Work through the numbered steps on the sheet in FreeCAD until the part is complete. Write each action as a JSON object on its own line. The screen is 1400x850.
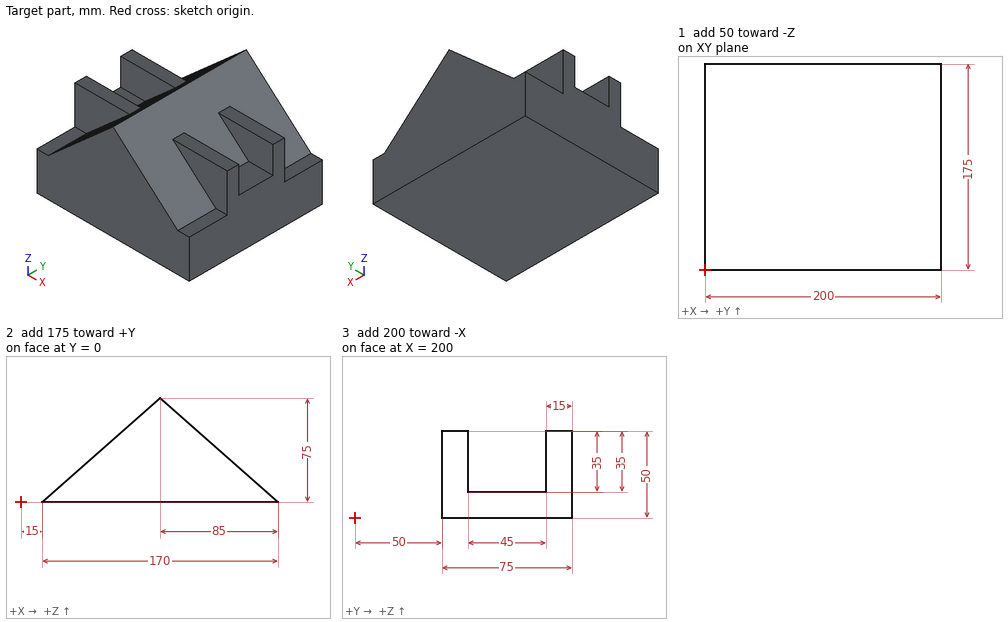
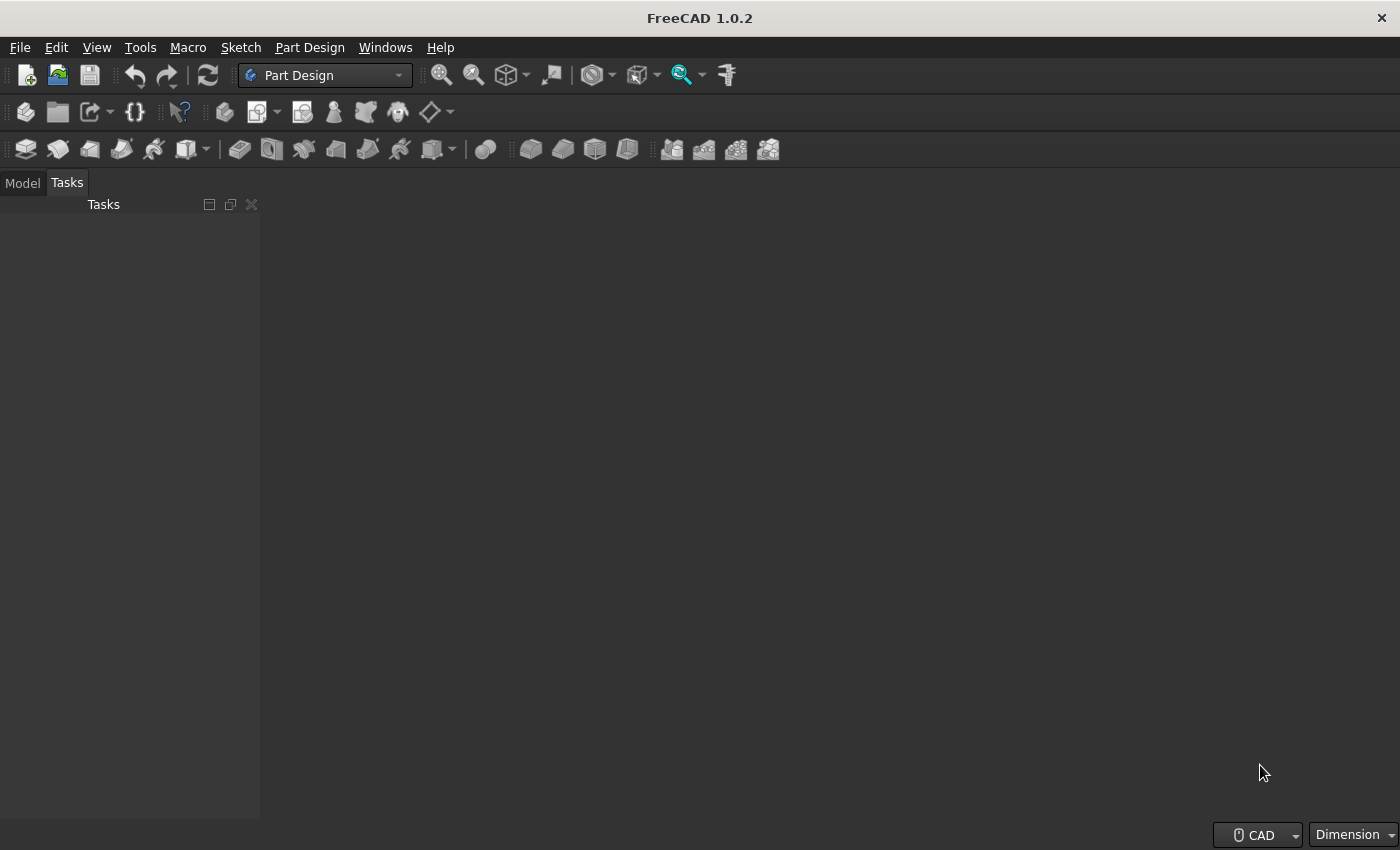
{"action": "left_click", "coordinate": [26, 76]}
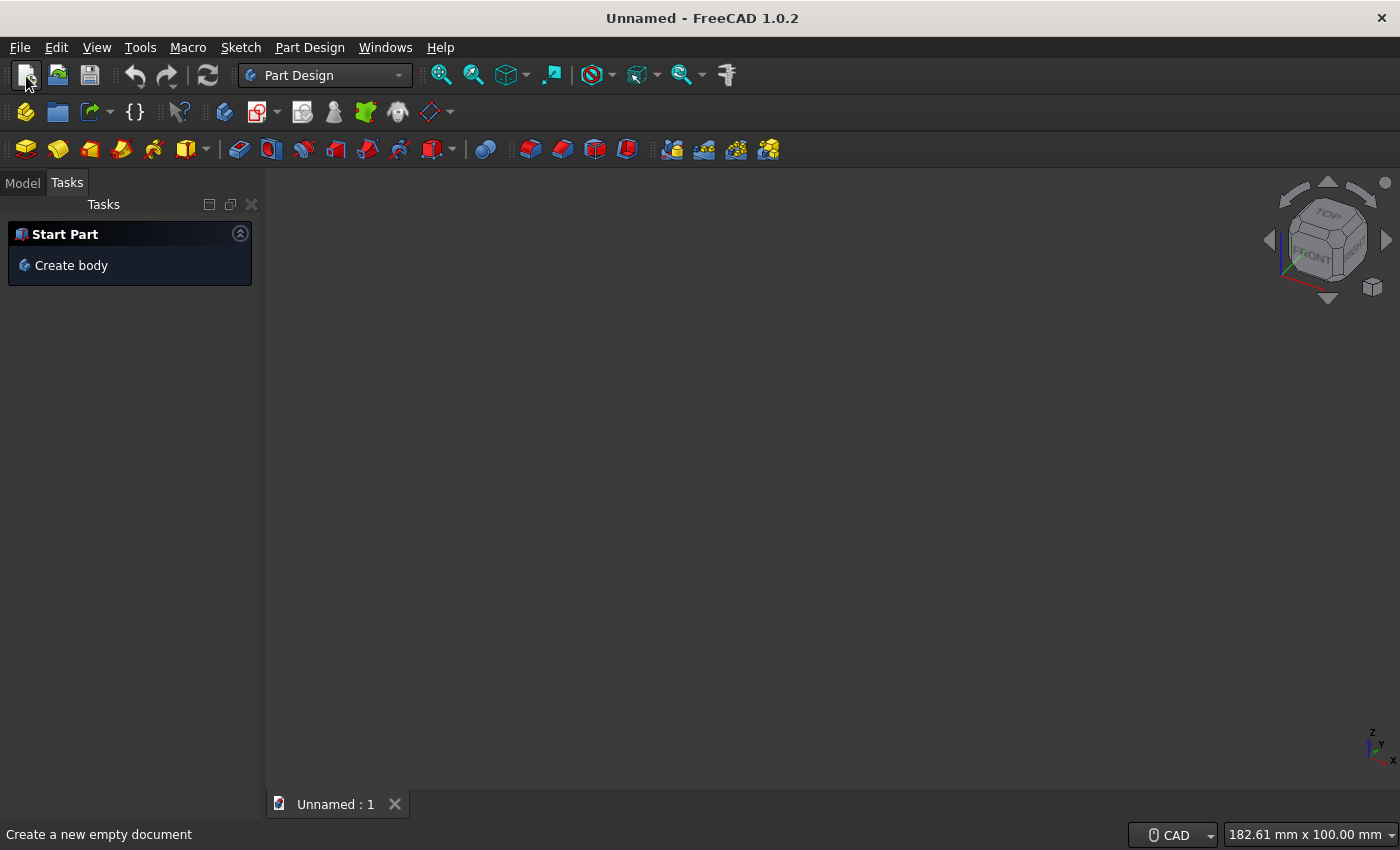
{"action": "left_click", "coordinate": [258, 112]}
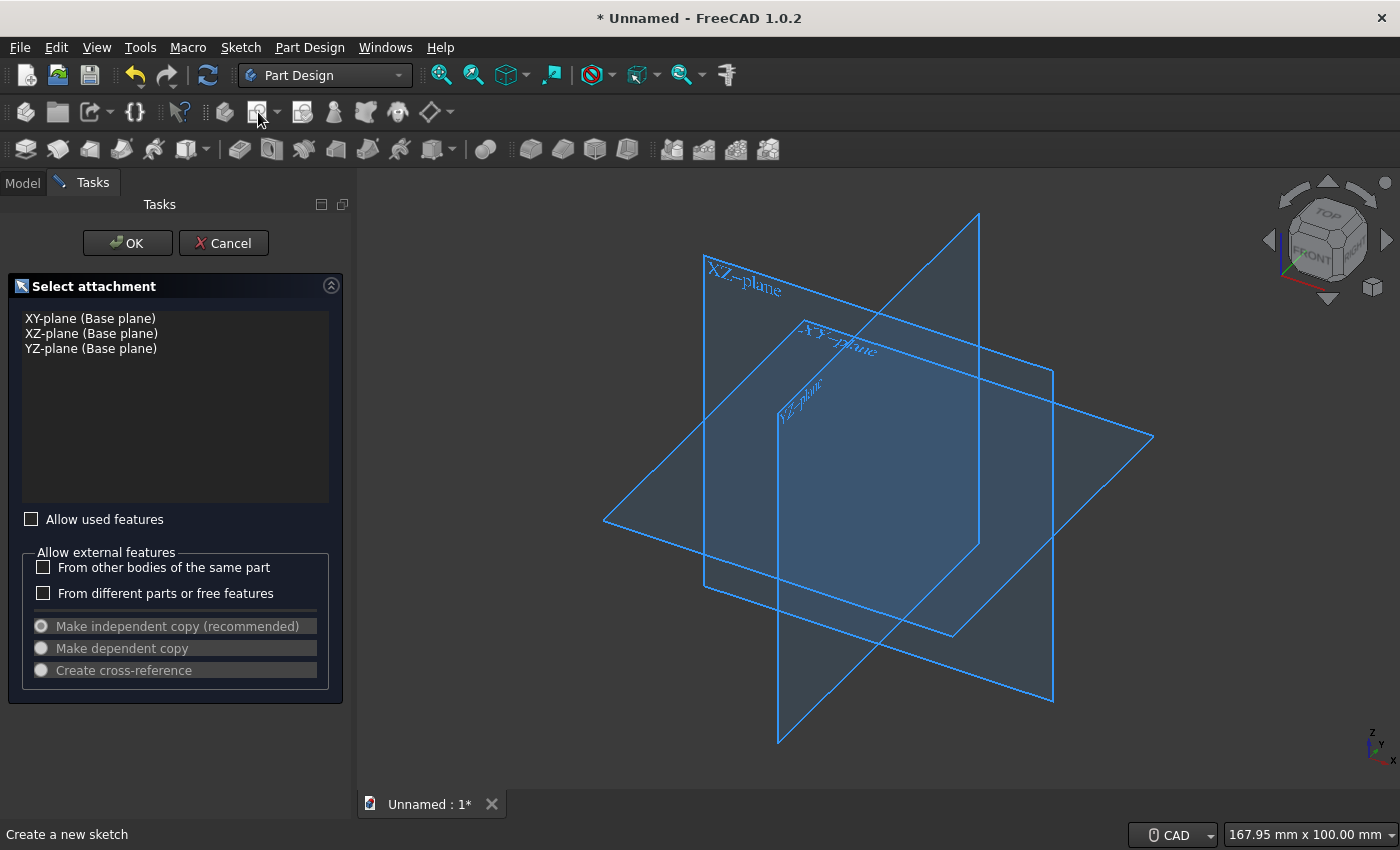
{"action": "left_click", "coordinate": [82, 318]}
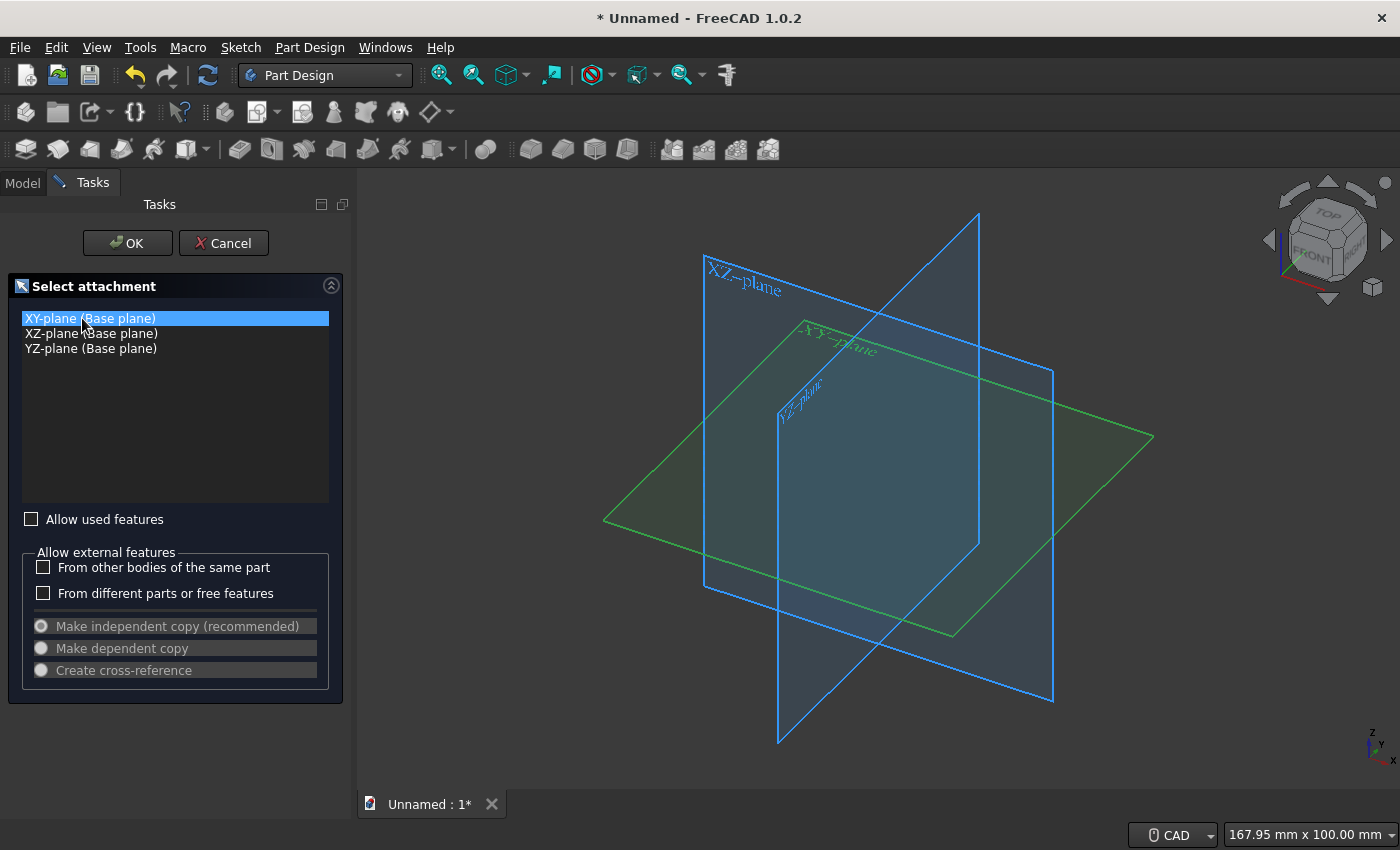
{"action": "left_click", "coordinate": [128, 243]}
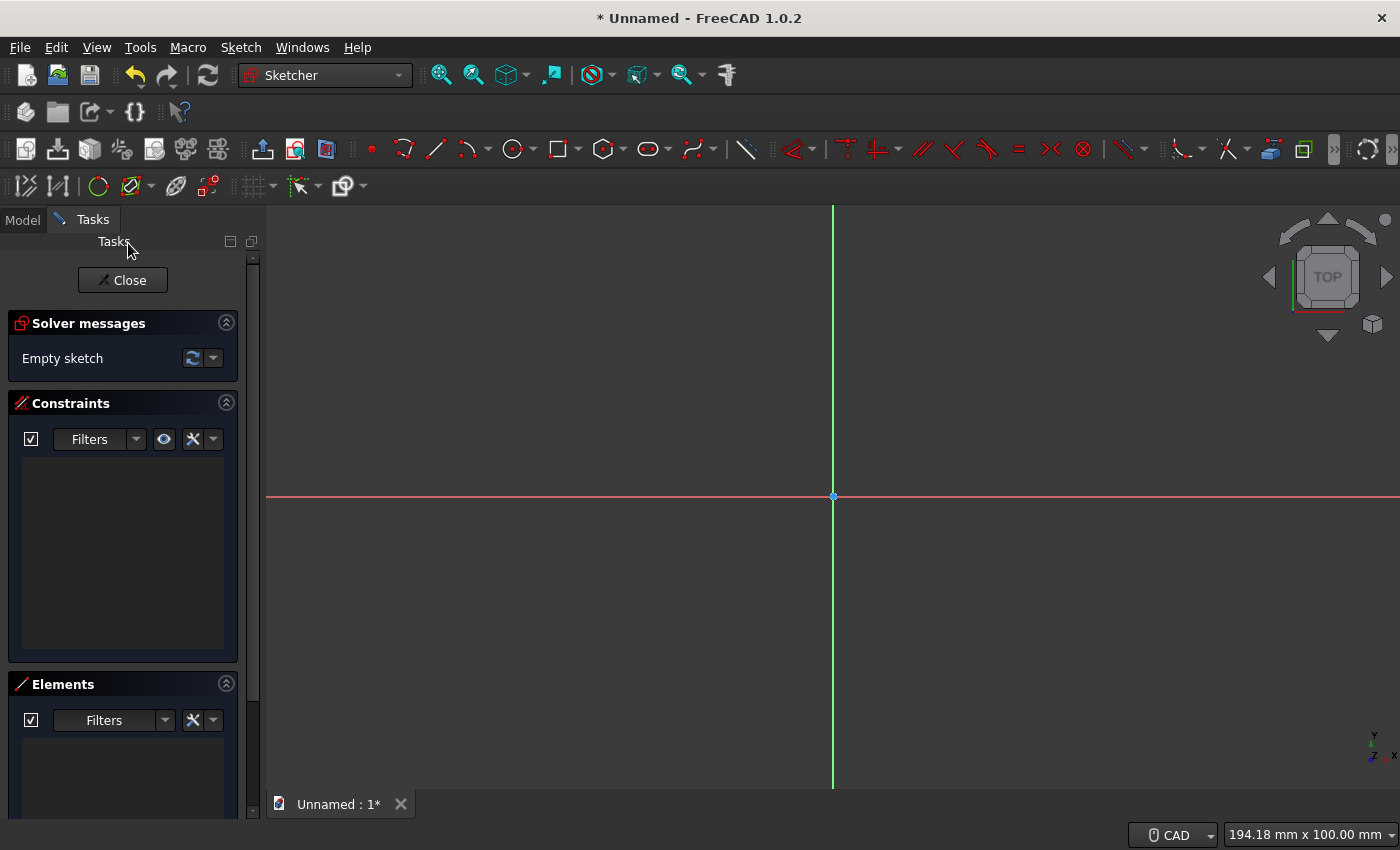
{"action": "scroll", "coordinate": [385, 761], "scroll_direction": "down", "scroll_amount": 5}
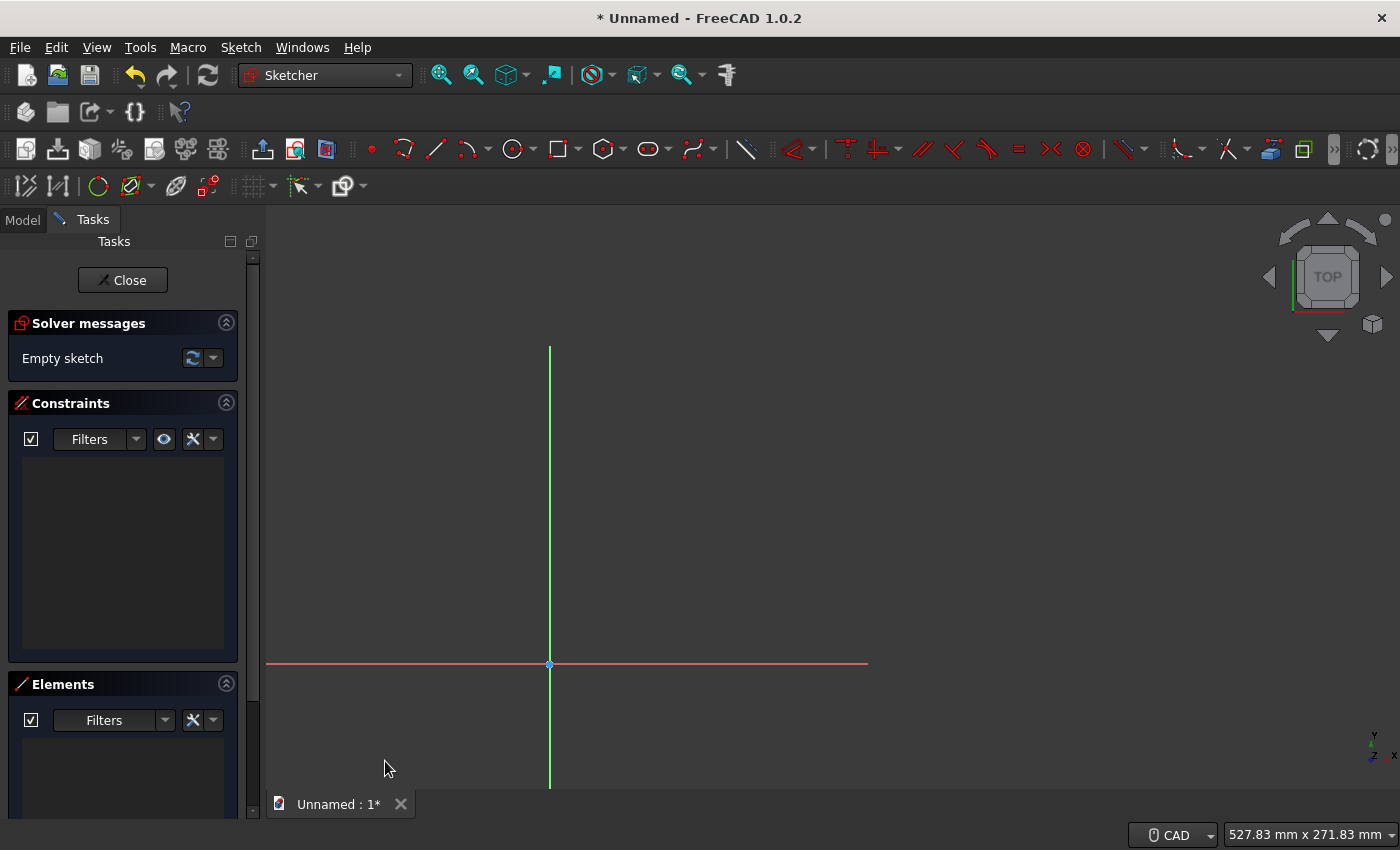
{"action": "left_click", "coordinate": [558, 150]}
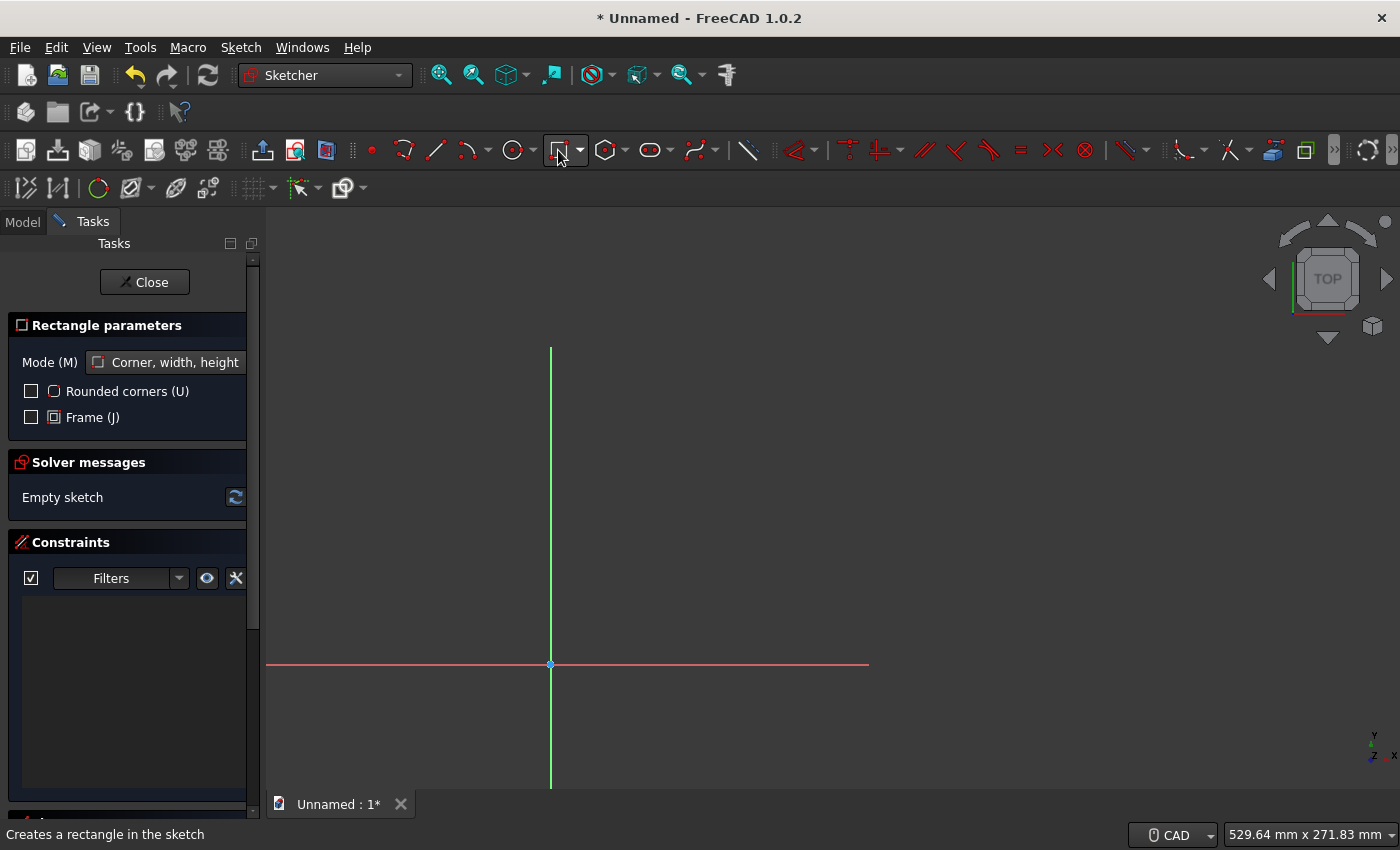
{"action": "left_click", "coordinate": [551, 665]}
{"action": "left_click", "coordinate": [979, 290]}
{"action": "key", "text": "Escape"}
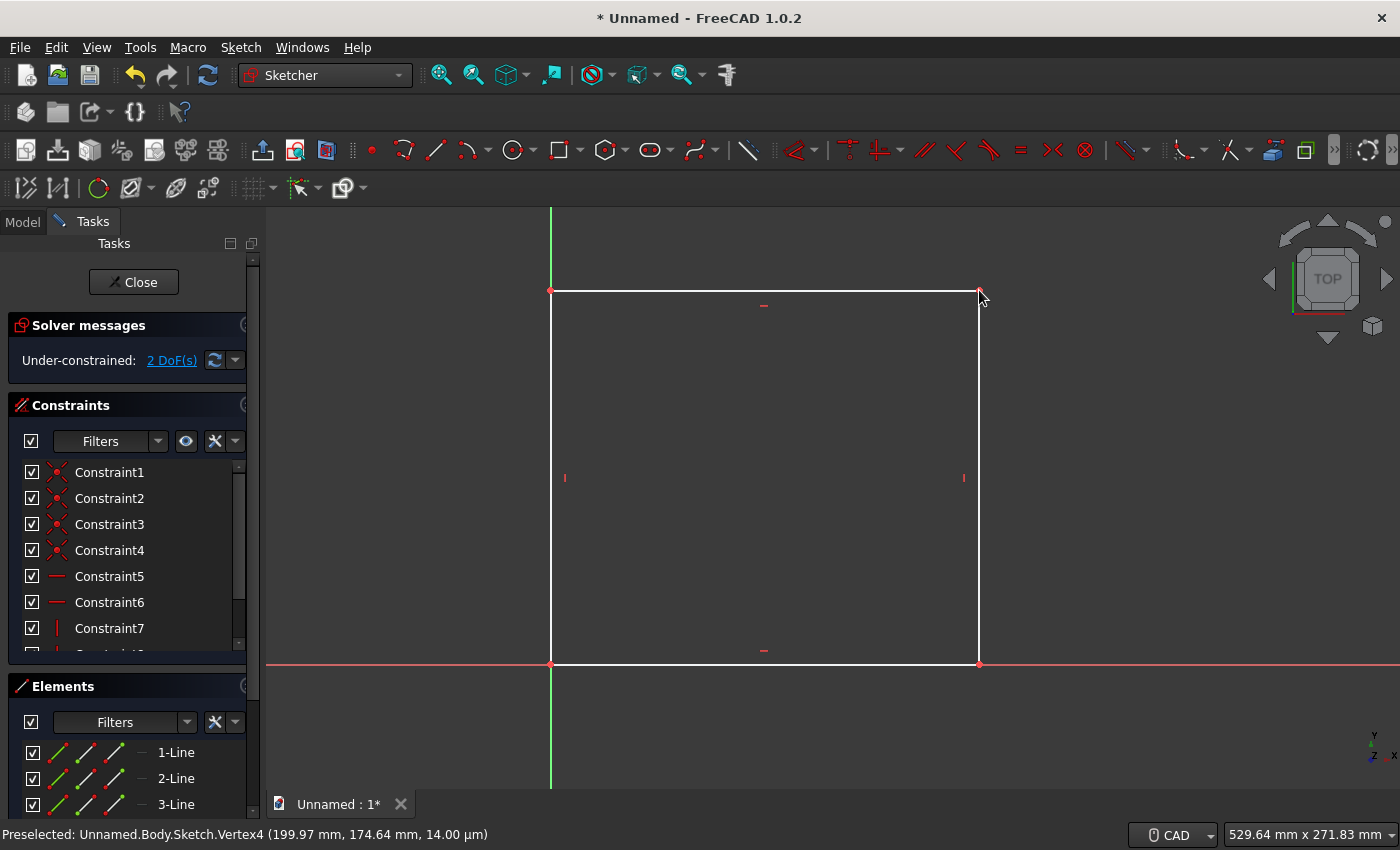
{"action": "left_click", "coordinate": [794, 150]}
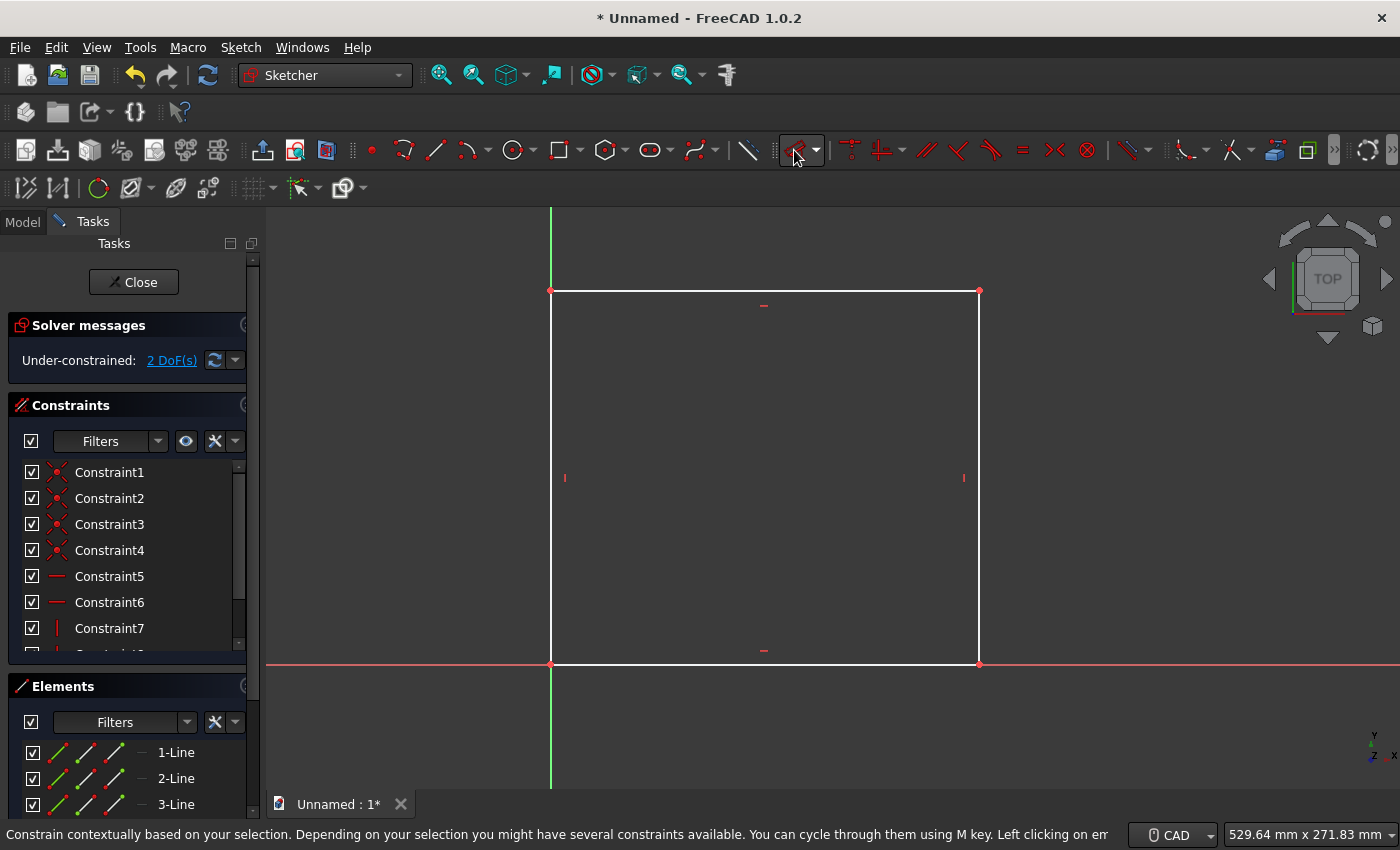
{"action": "left_click", "coordinate": [679, 665]}
{"action": "left_click", "coordinate": [765, 699]}